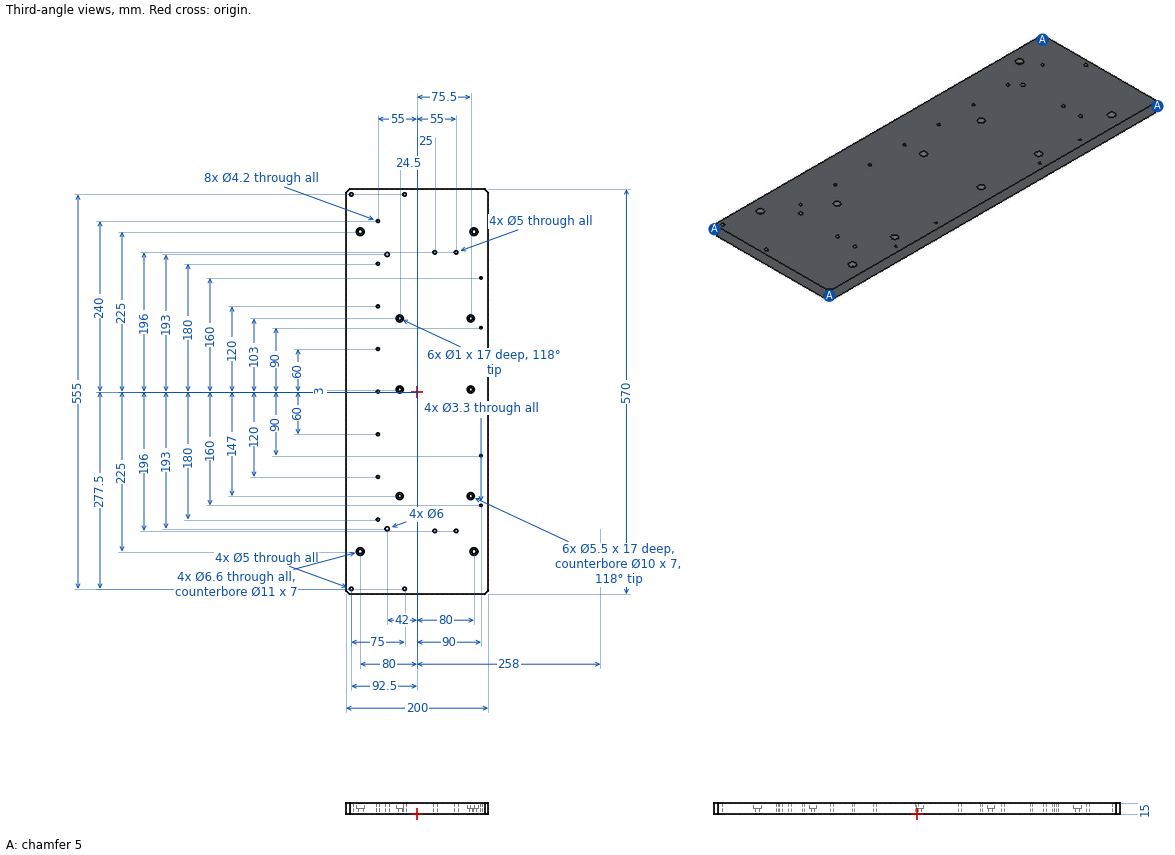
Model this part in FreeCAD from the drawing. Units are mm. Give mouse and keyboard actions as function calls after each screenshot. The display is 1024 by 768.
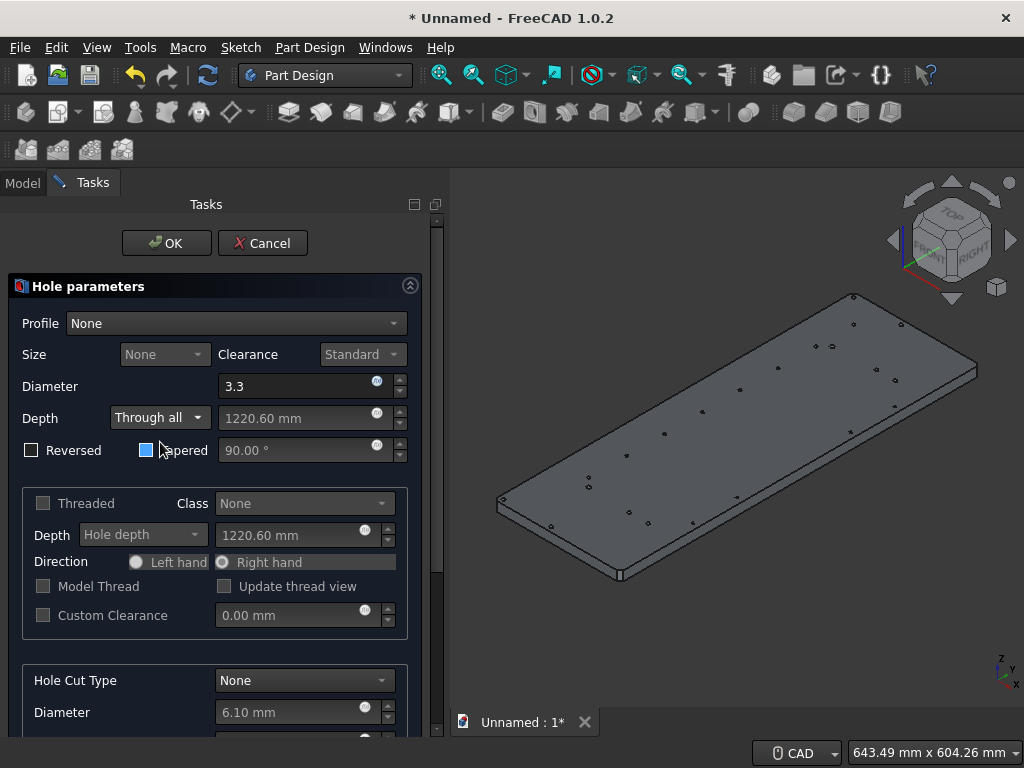
click(167, 243)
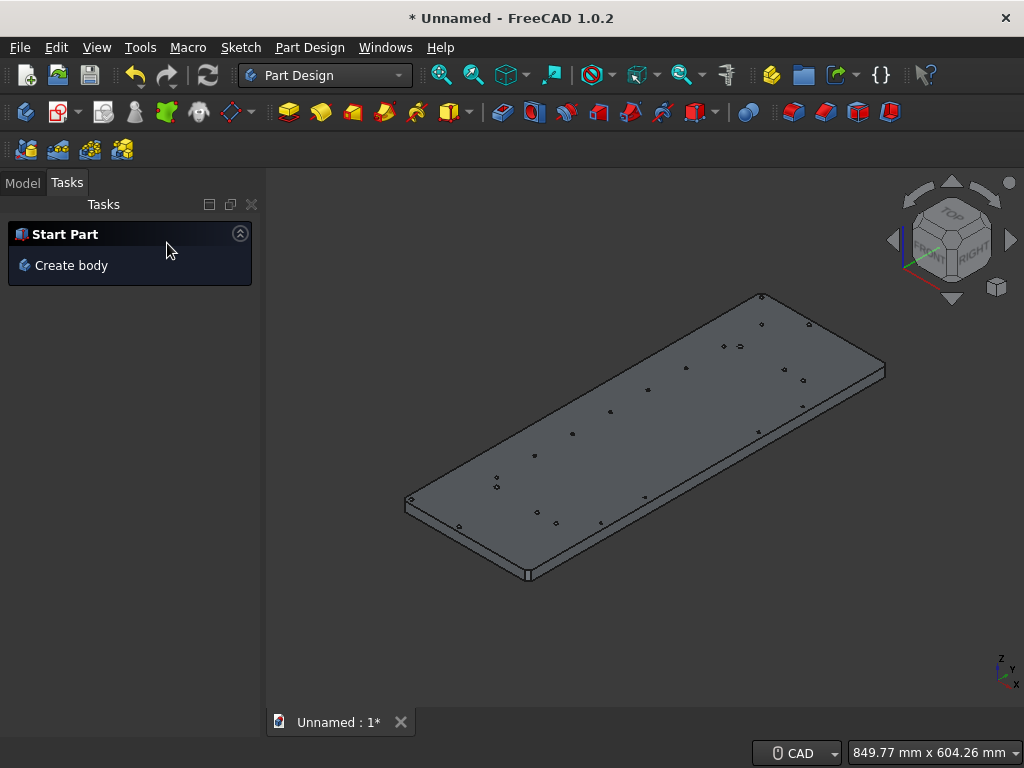
key(5)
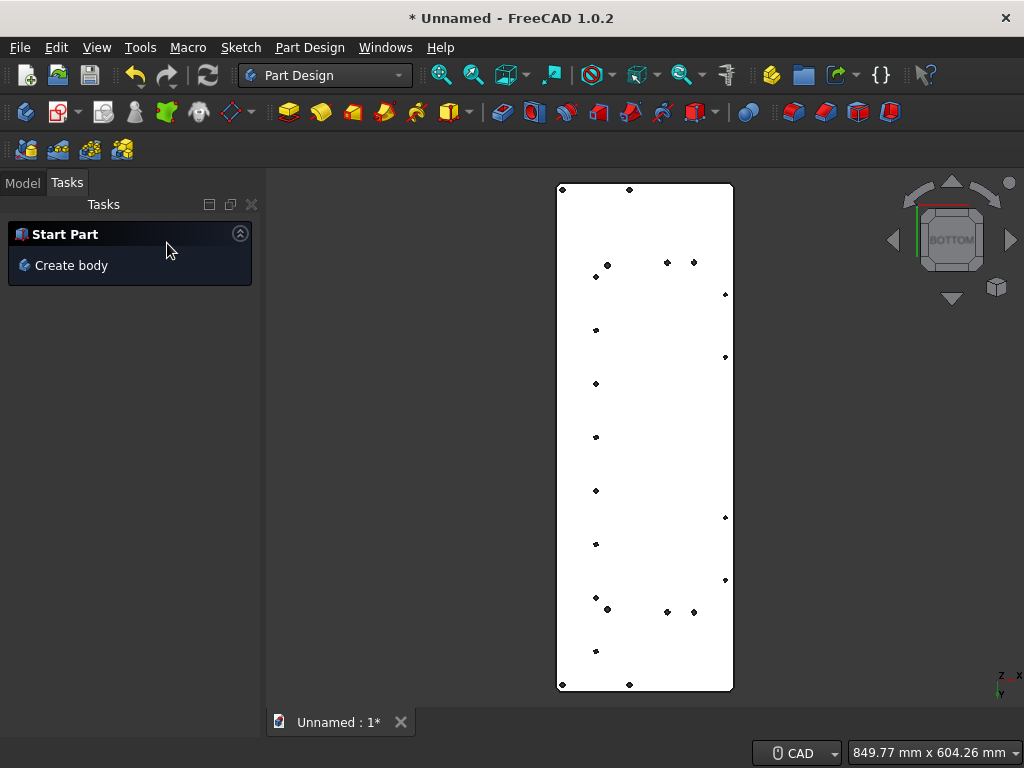
click(670, 437)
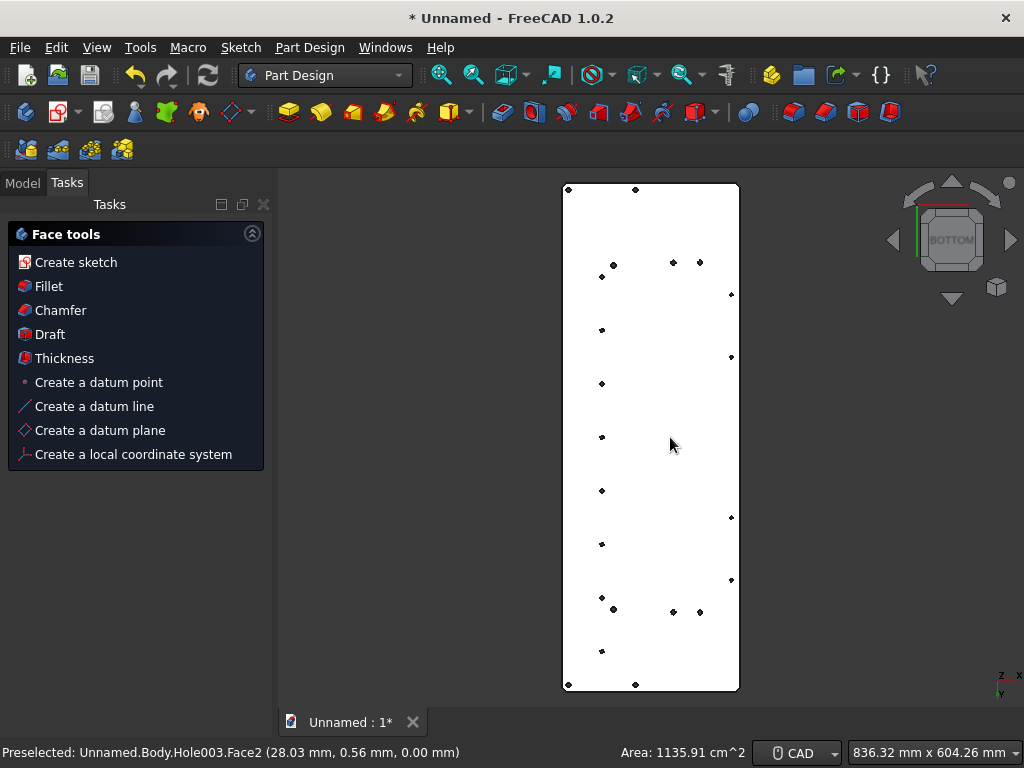
click(58, 112)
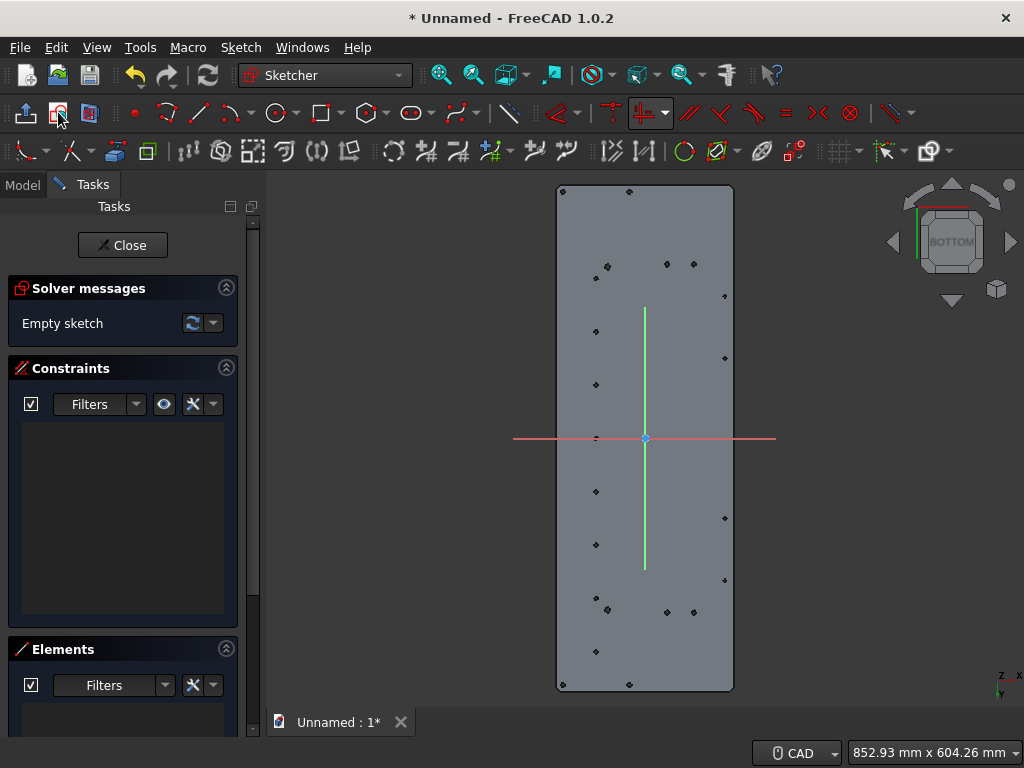
scroll(853, 379, up, 2)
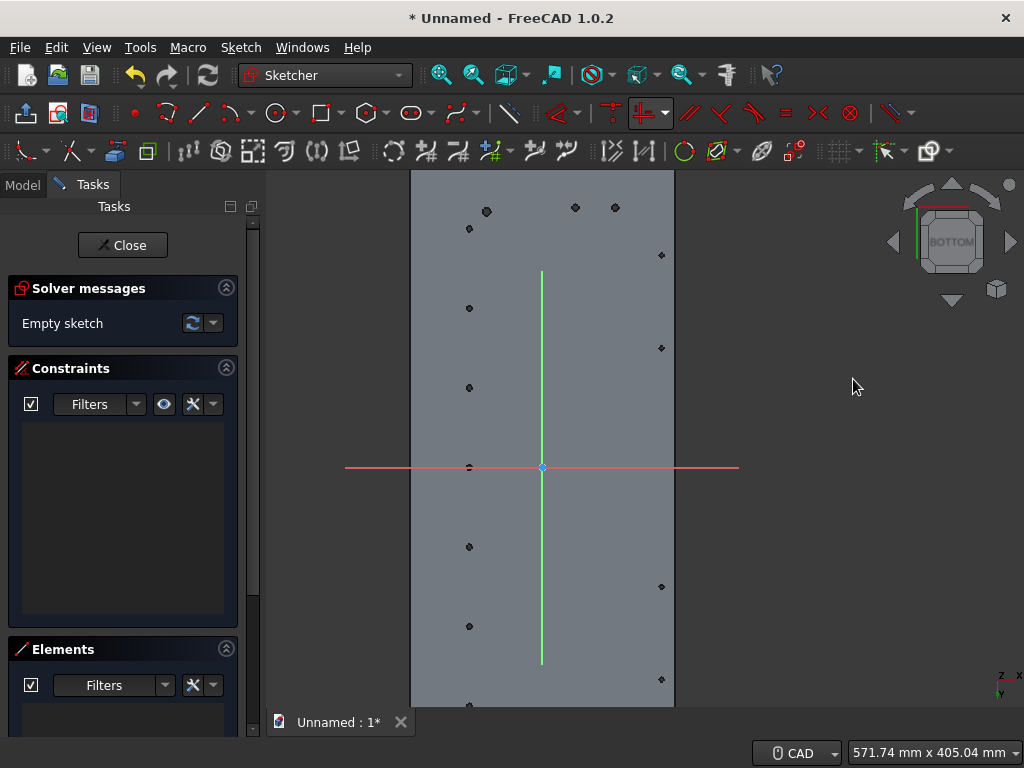
click(276, 114)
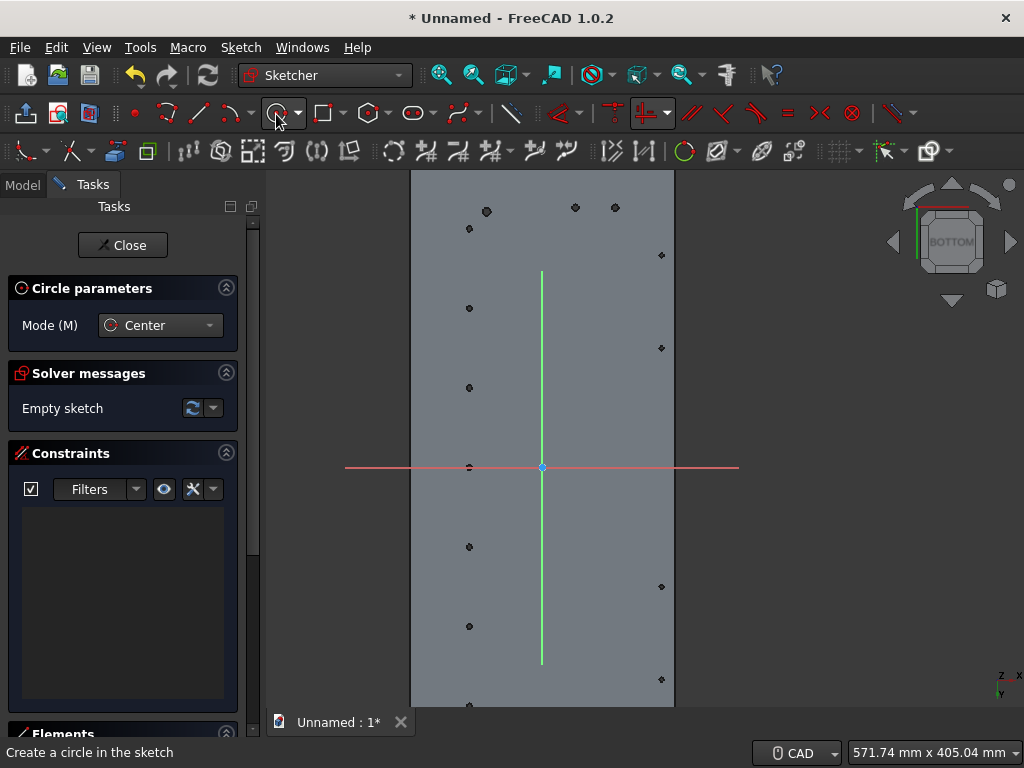
scroll(510, 604, up, 18)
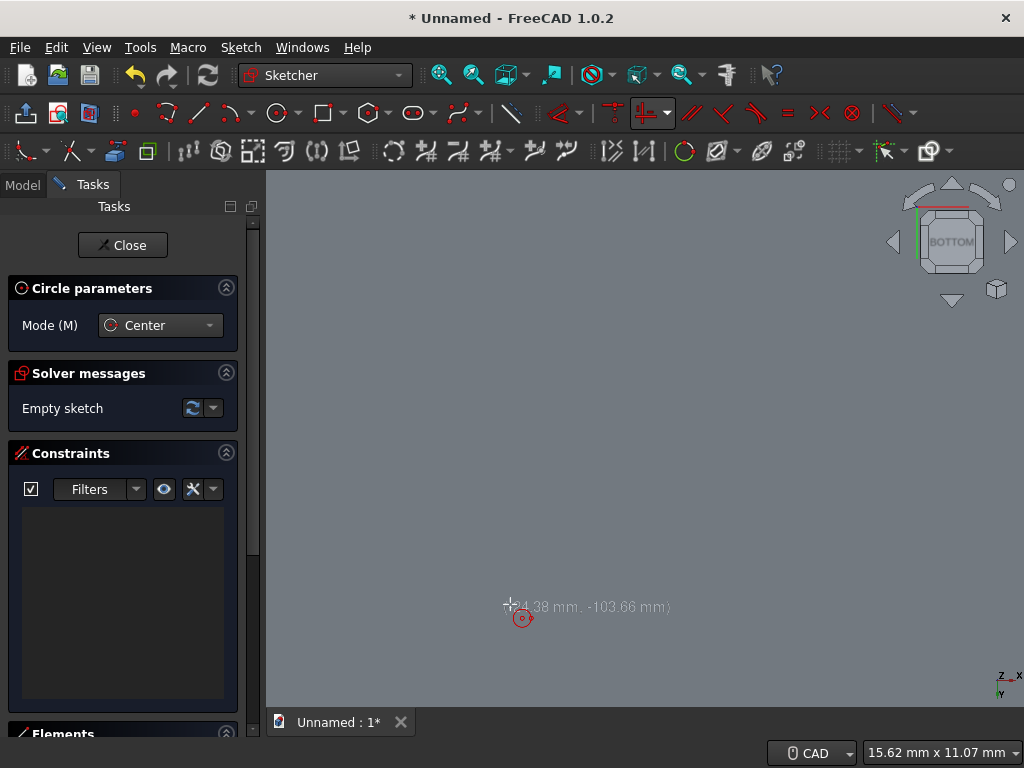
scroll(496, 643, down, 17)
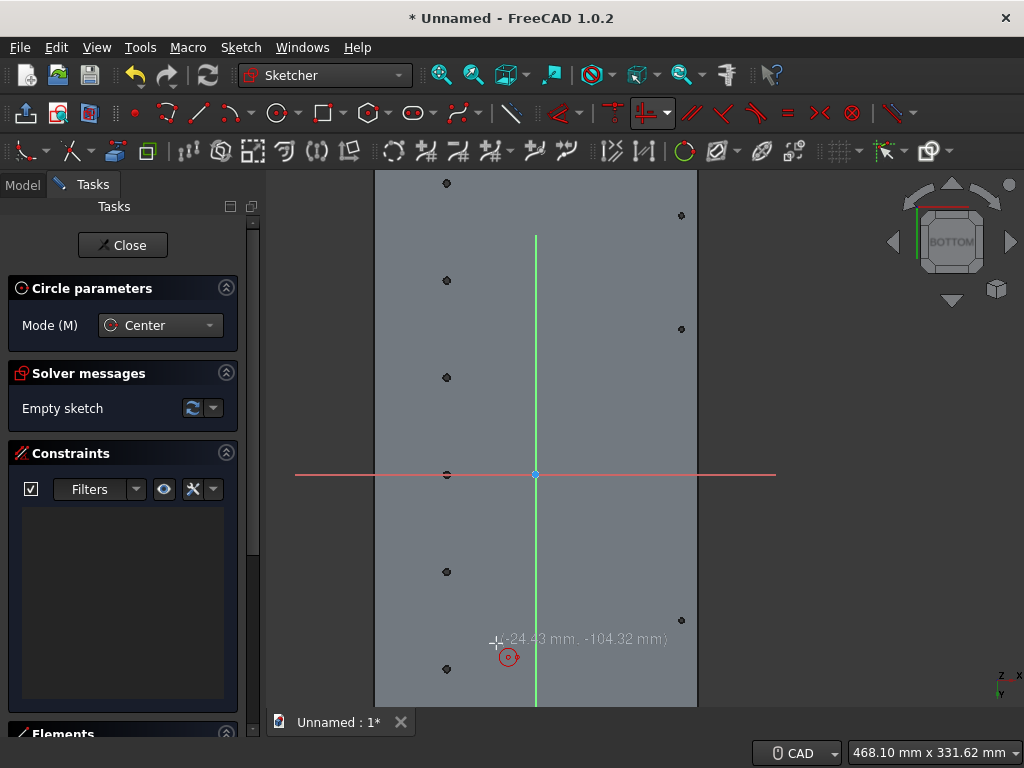
click(496, 642)
move(497, 641)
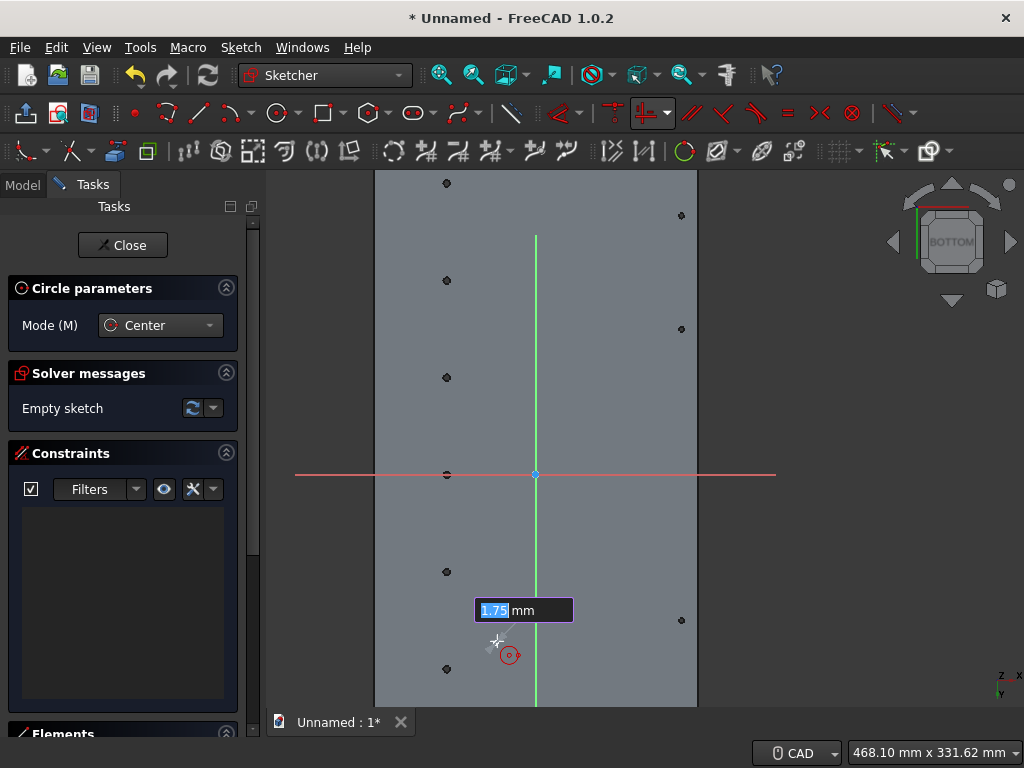
text(1)
key(Return)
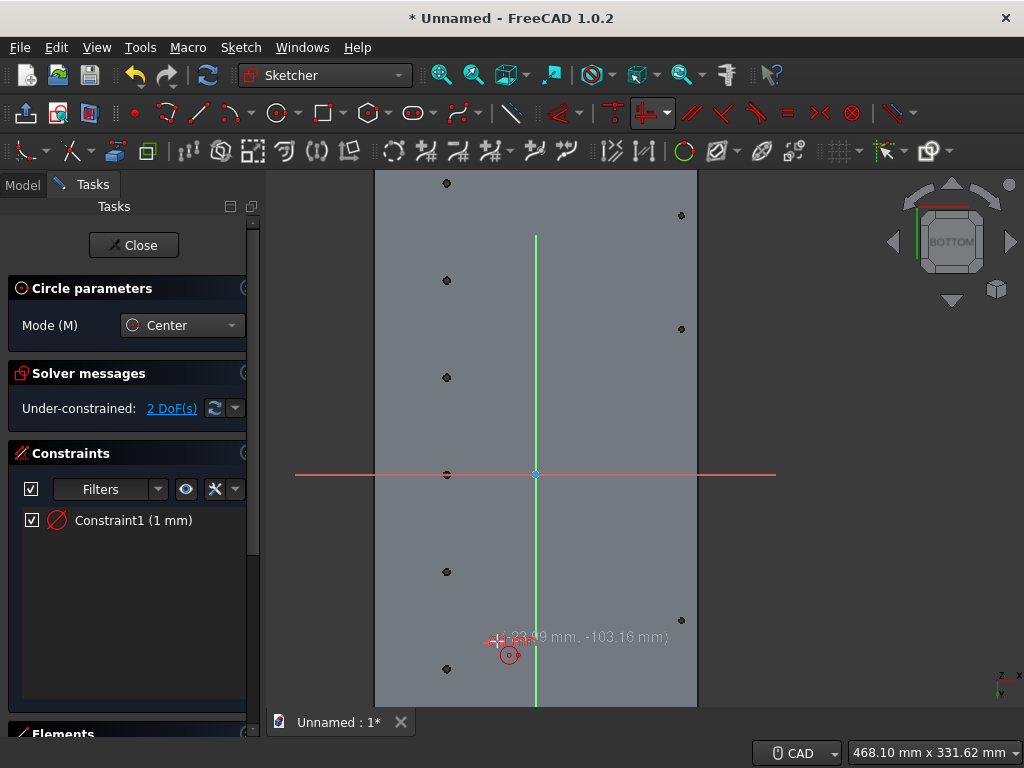
scroll(658, 642, up, 17)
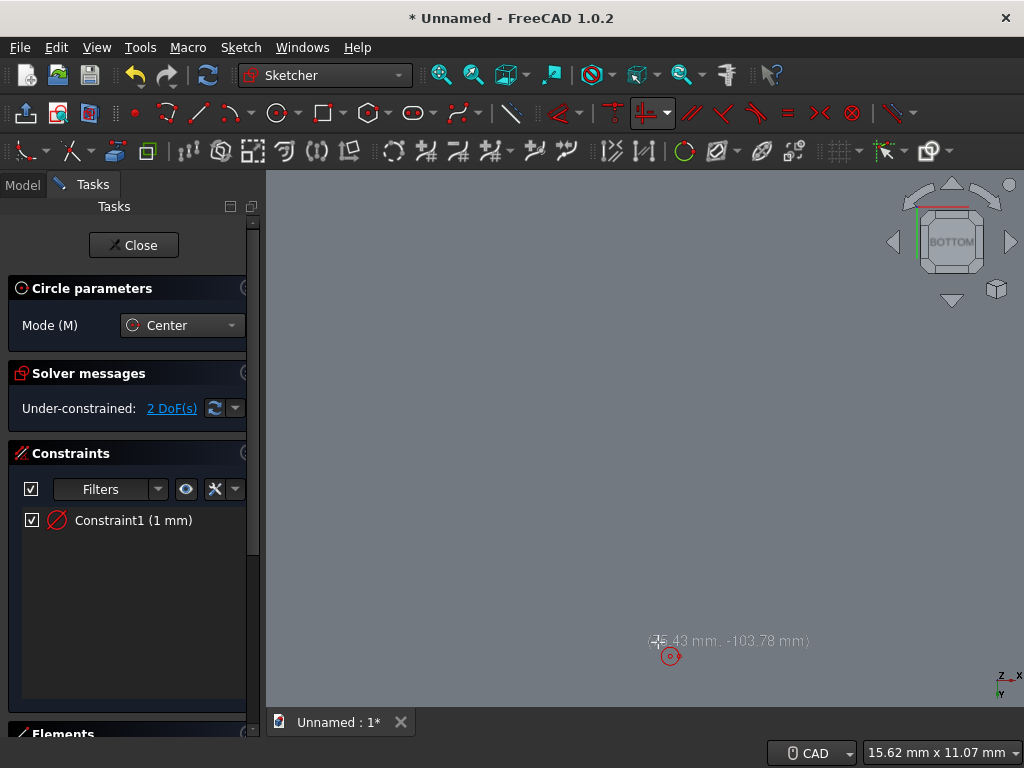
scroll(658, 642, down, 17)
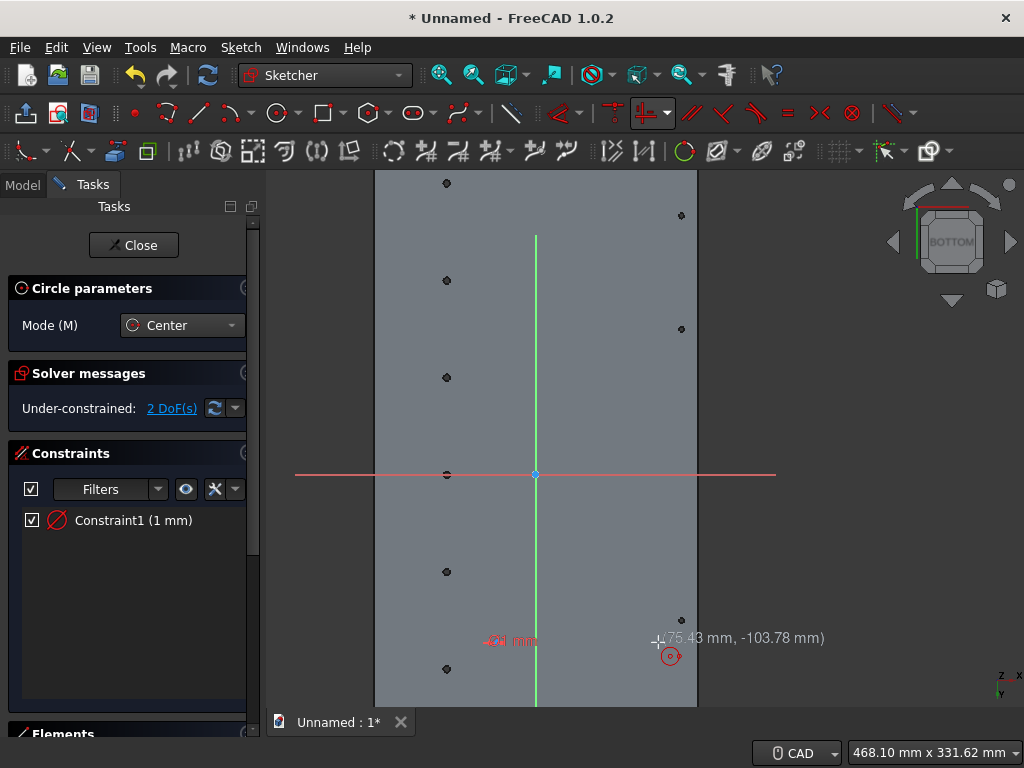
click(658, 642)
move(659, 641)